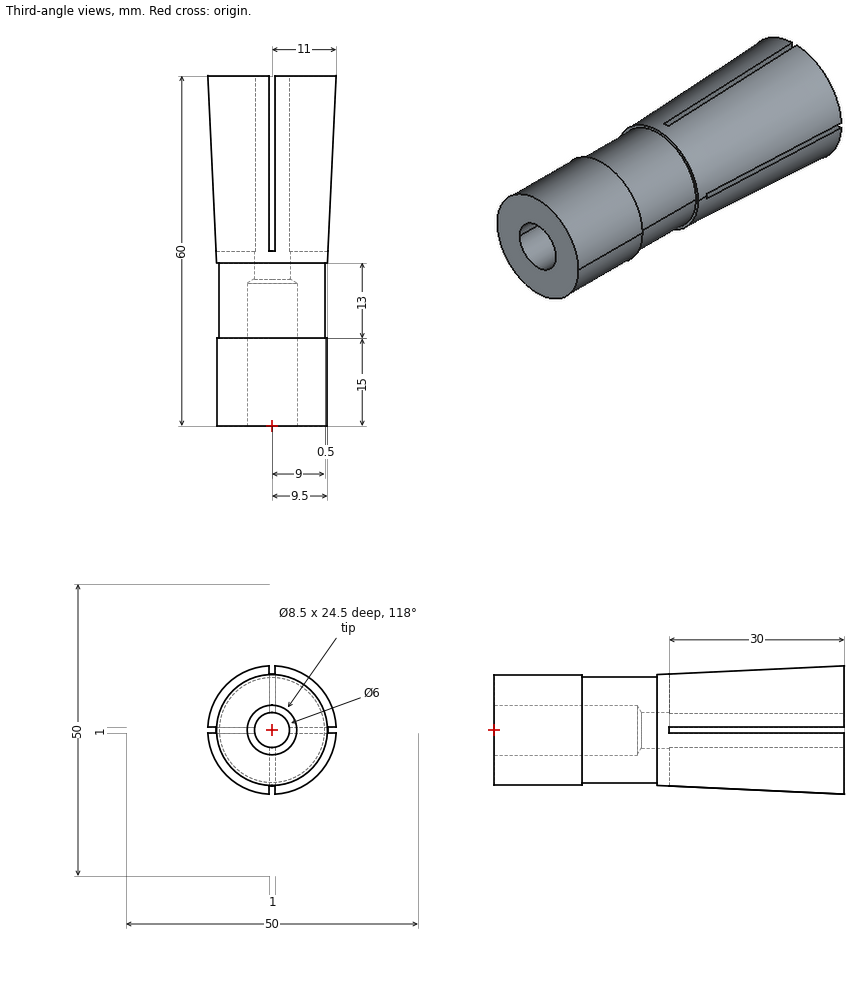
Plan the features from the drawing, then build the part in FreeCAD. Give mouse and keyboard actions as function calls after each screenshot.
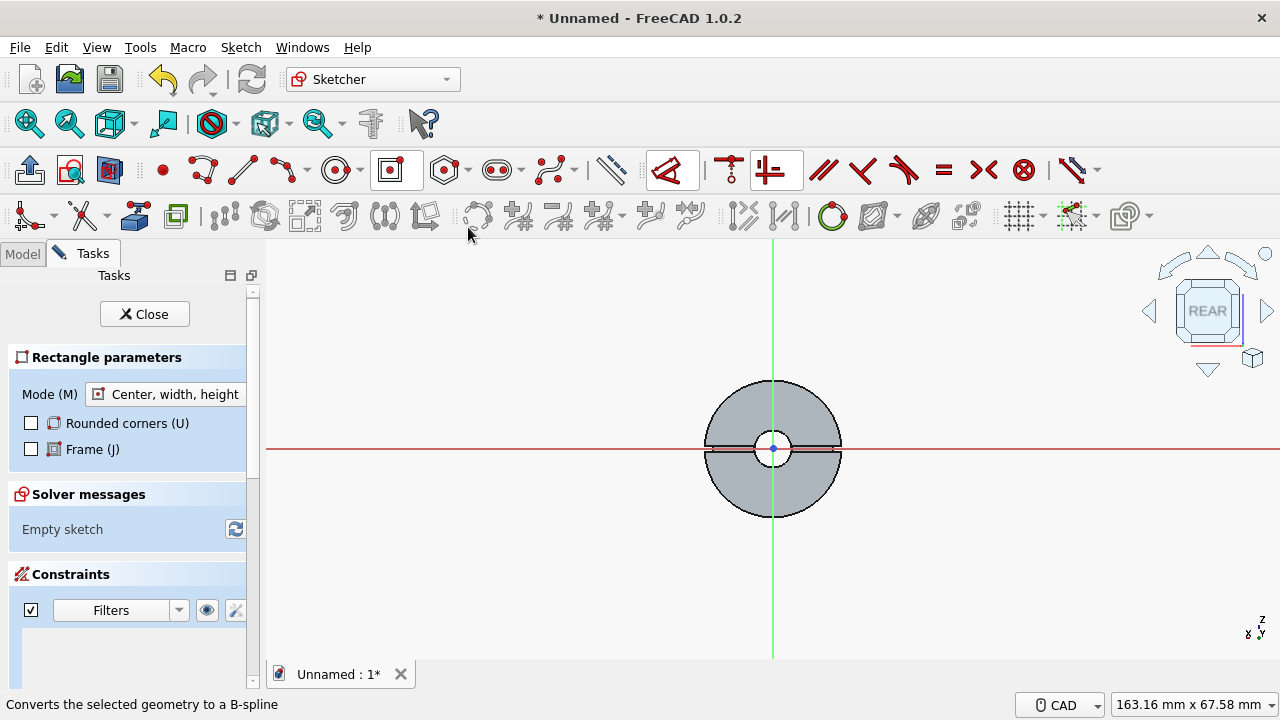
scroll(773, 449, up, 9)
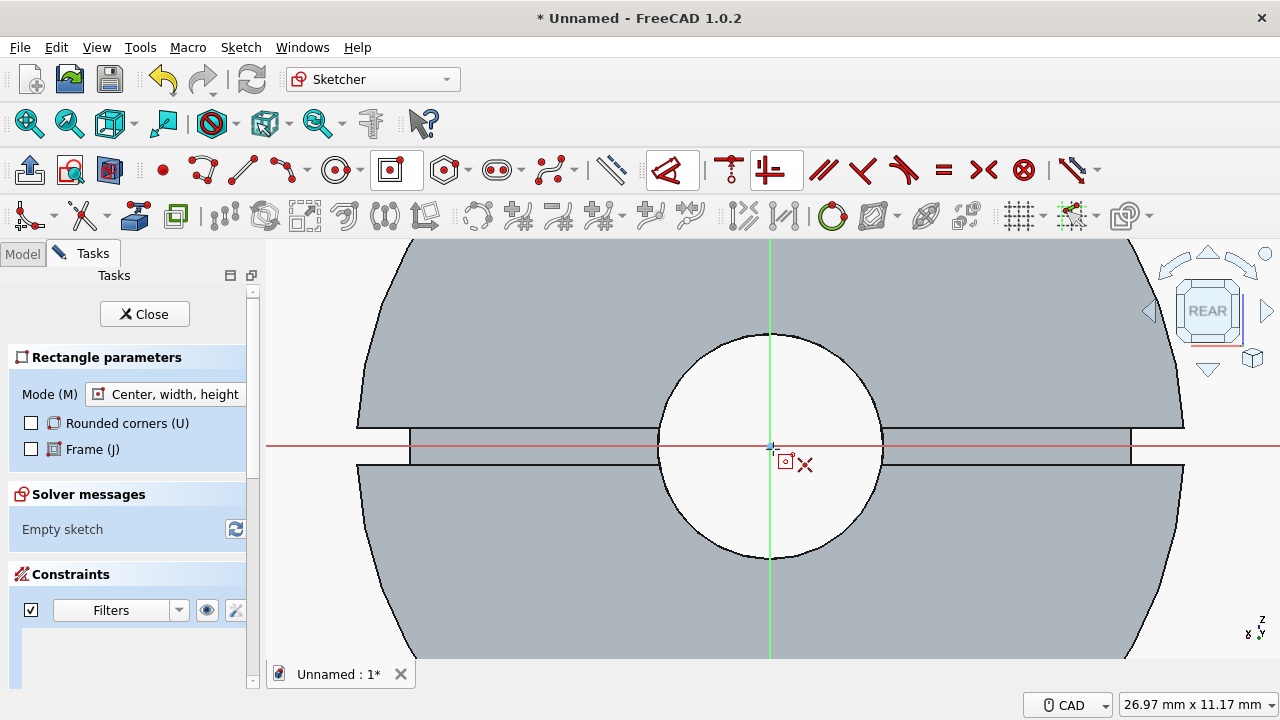
scroll(694, 449, down, 10)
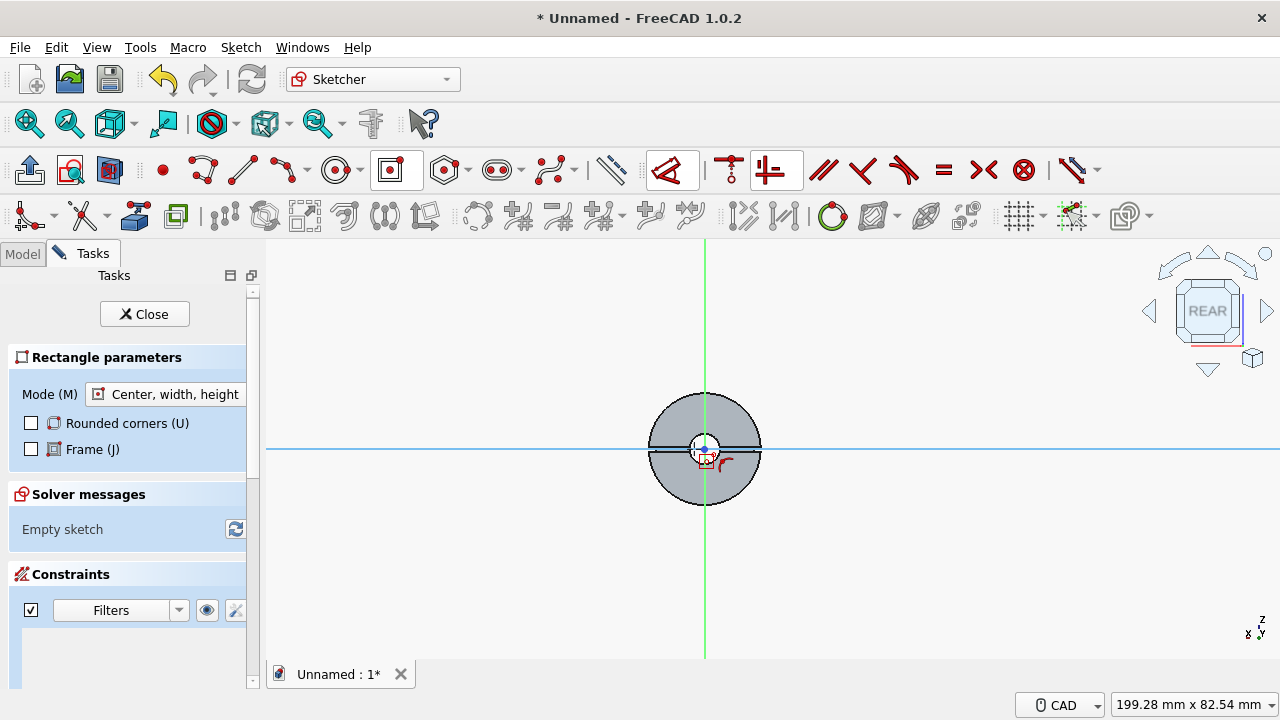
click(705, 449)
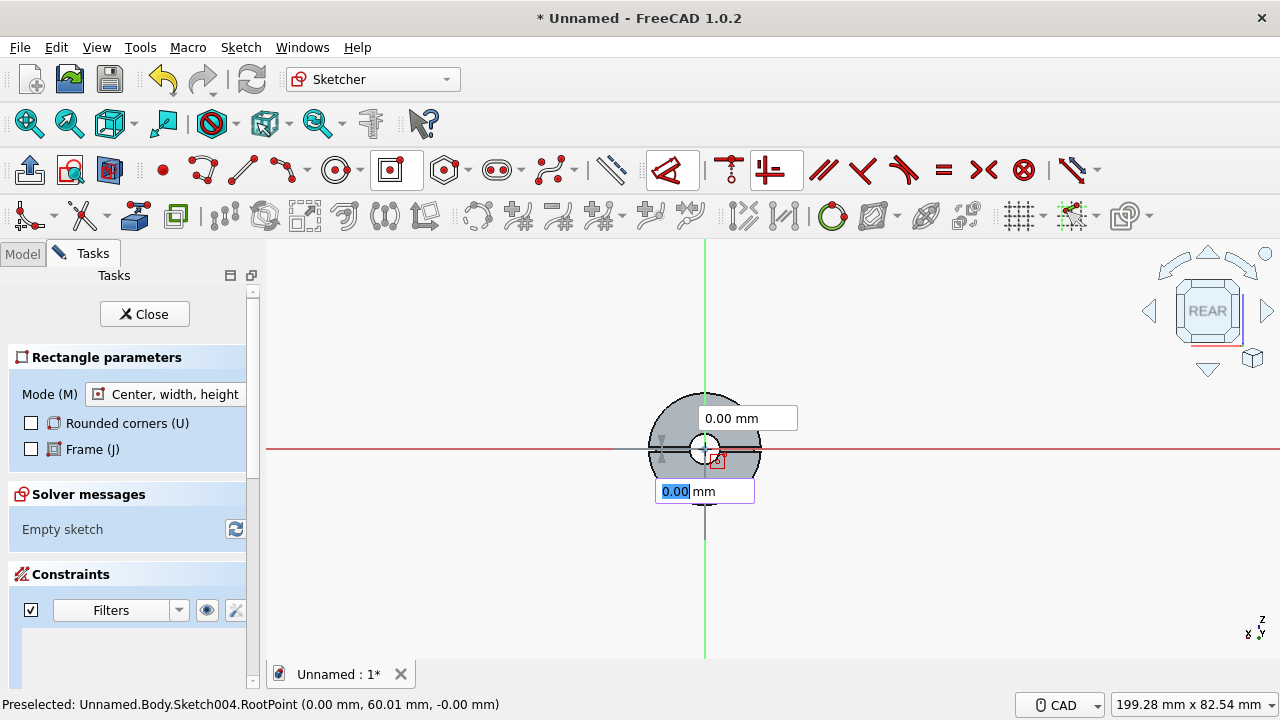
scroll(707, 322, up, 10)
move(706, 320)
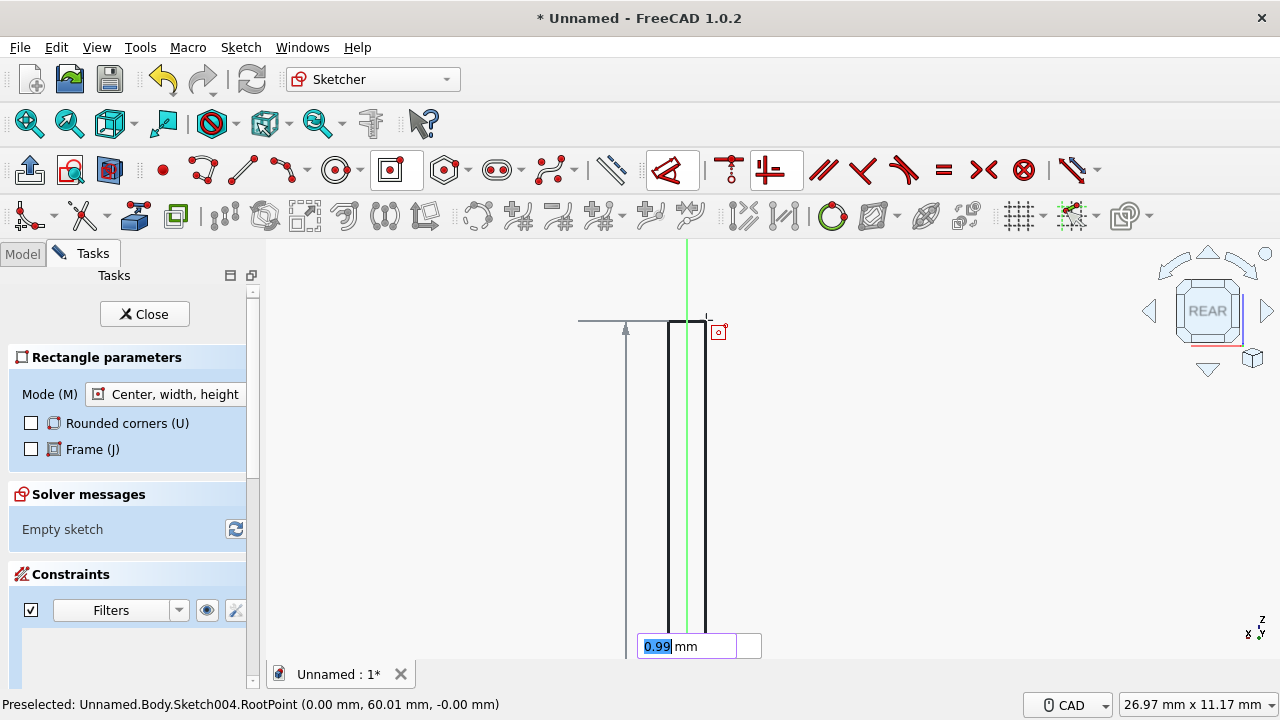
text(1)
key(Tab)
text(50)
key(Return)
key(Escape)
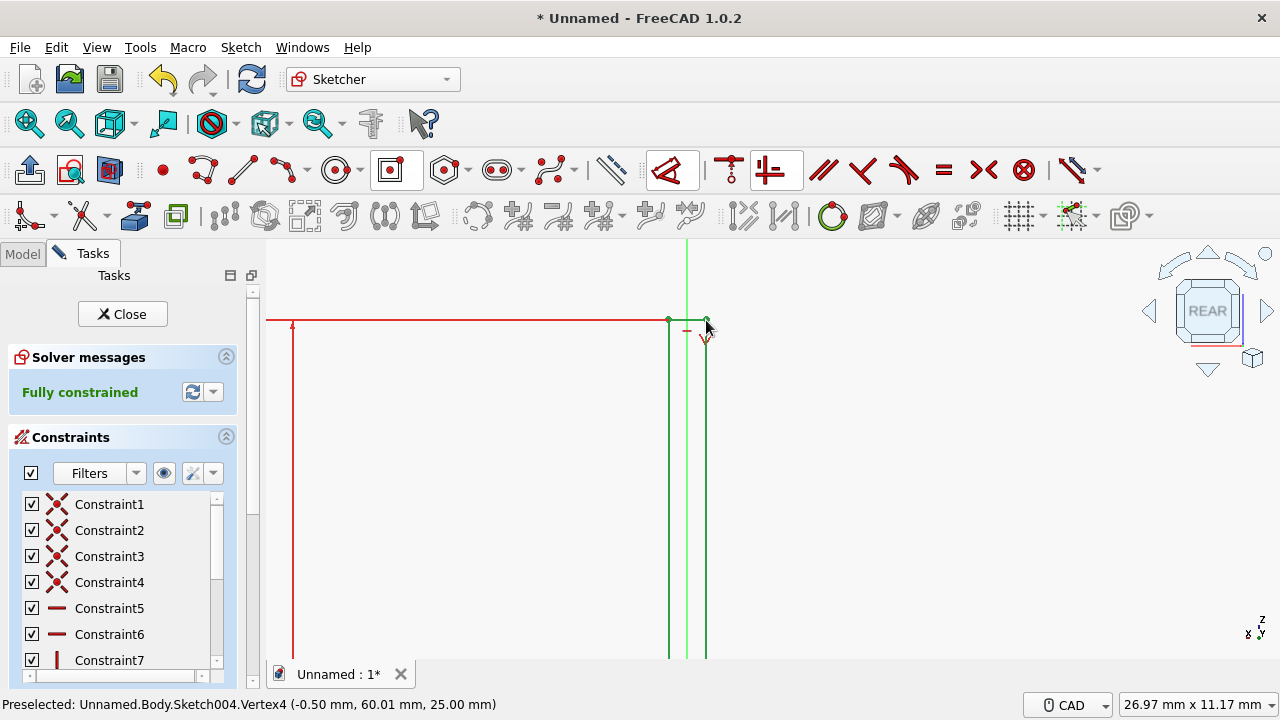
click(123, 314)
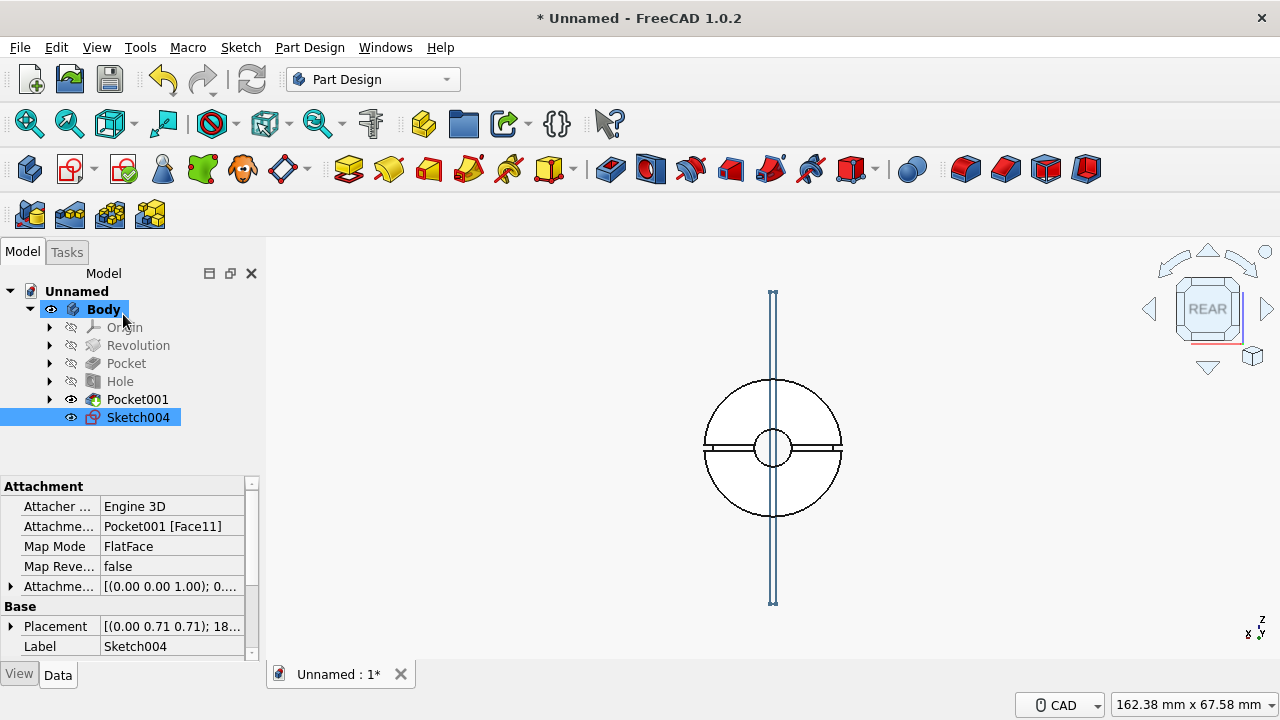
click(612, 170)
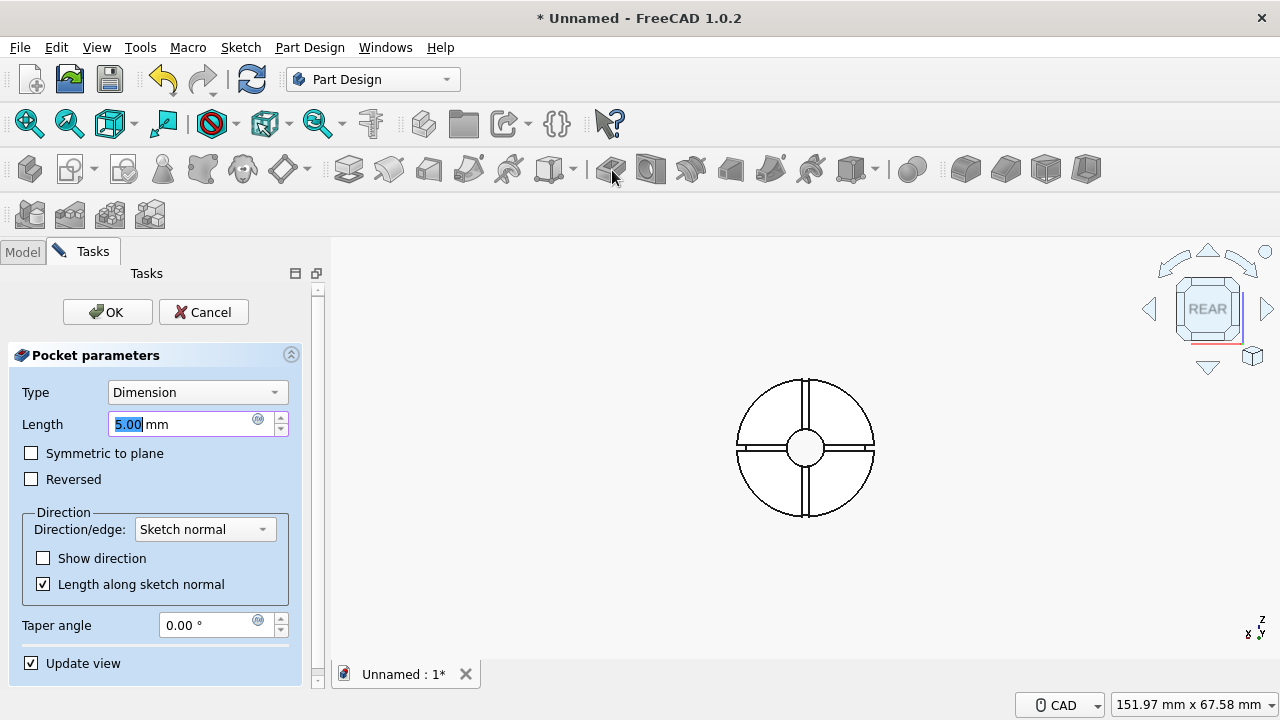
text(30)
key(Tab)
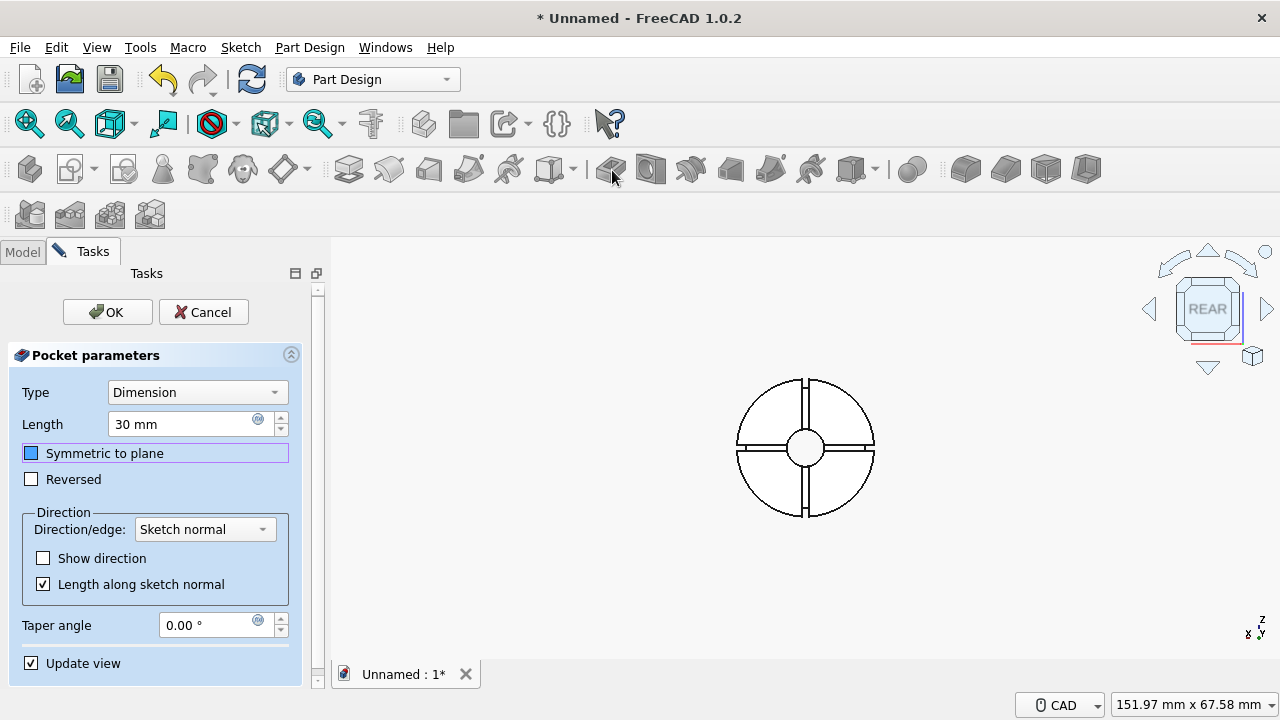
click(108, 312)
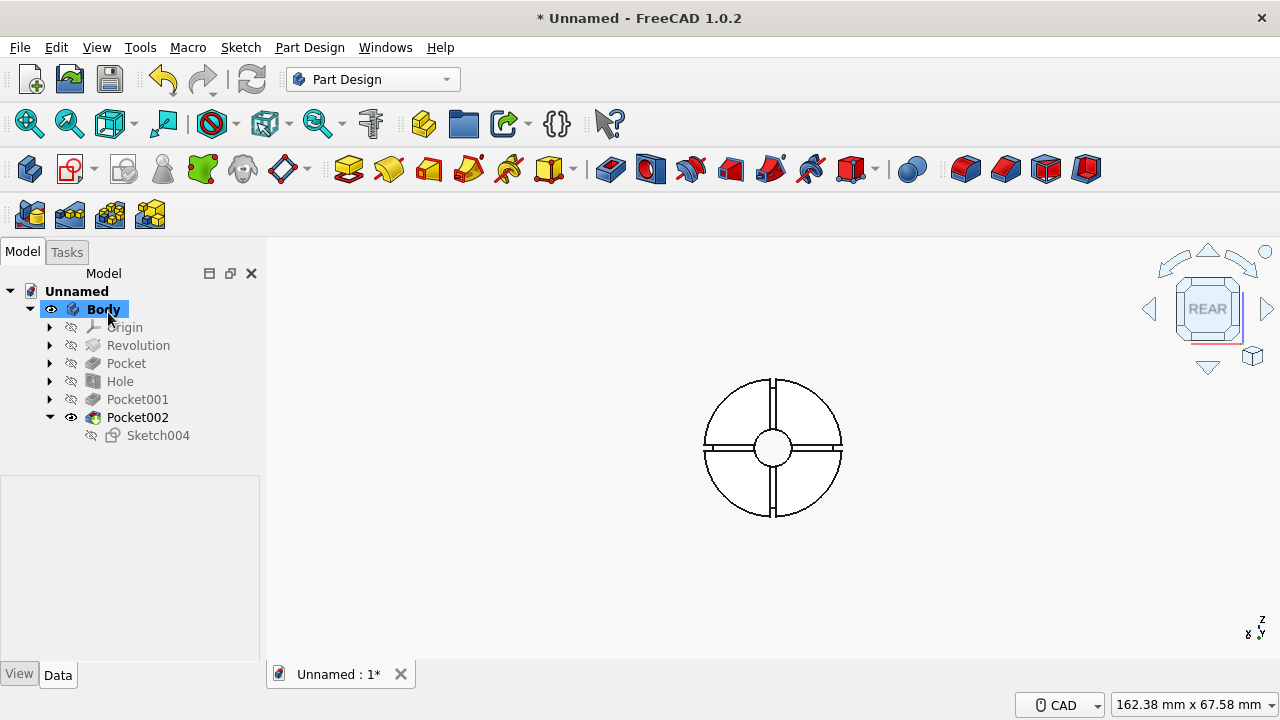
key(0)